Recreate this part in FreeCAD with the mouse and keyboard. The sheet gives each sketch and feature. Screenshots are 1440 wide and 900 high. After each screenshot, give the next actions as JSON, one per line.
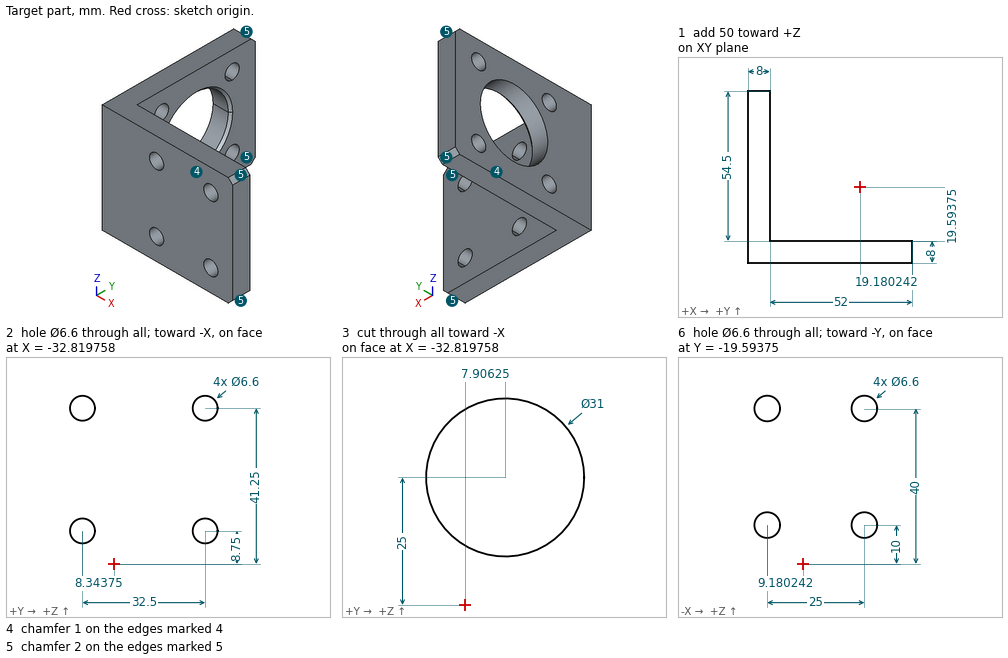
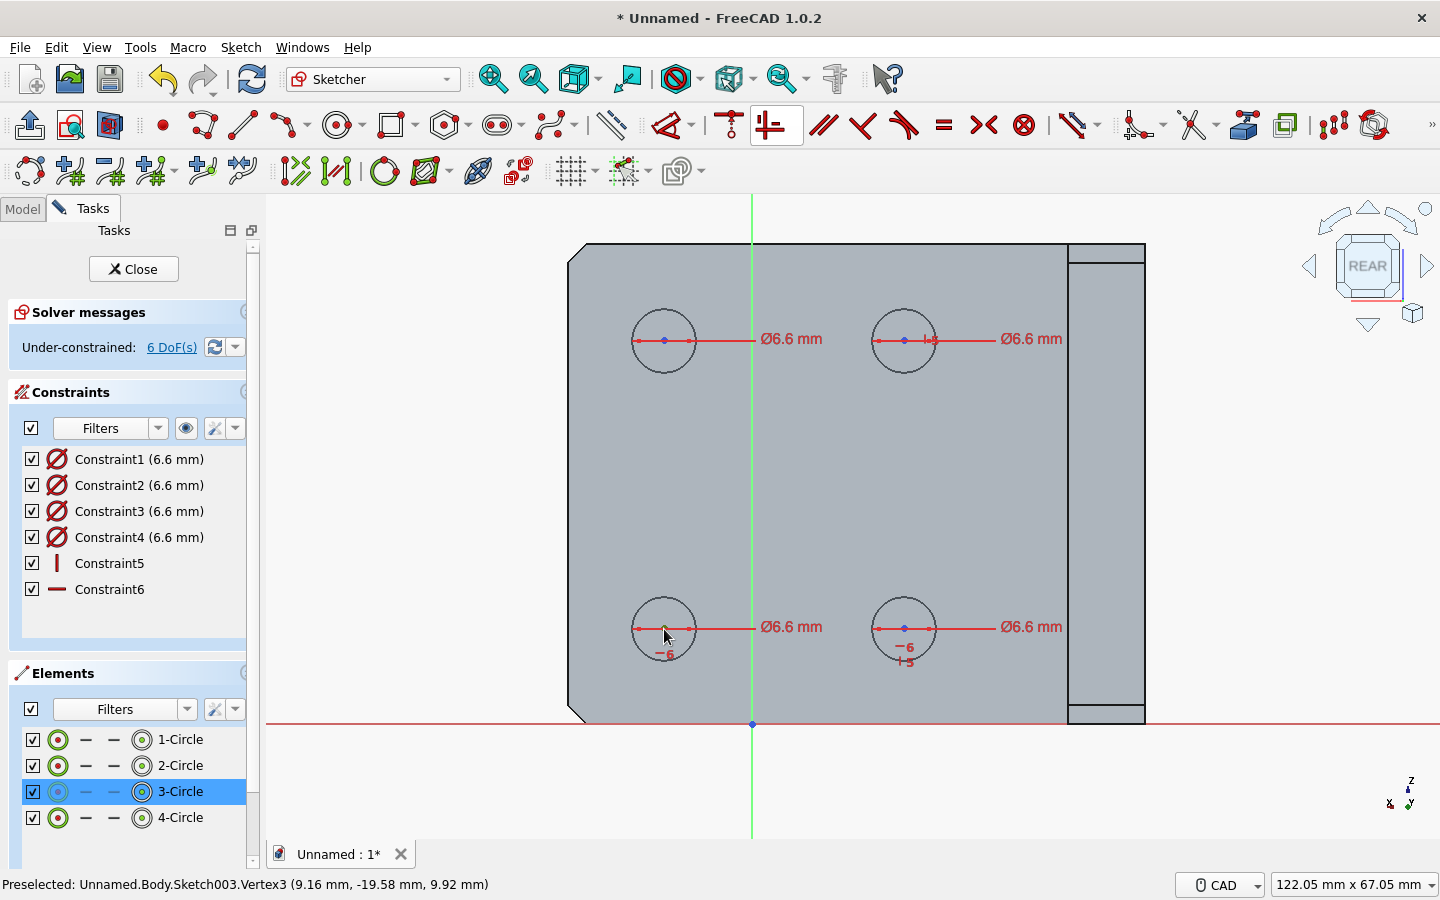
{"action": "left_click", "coordinate": [664, 341]}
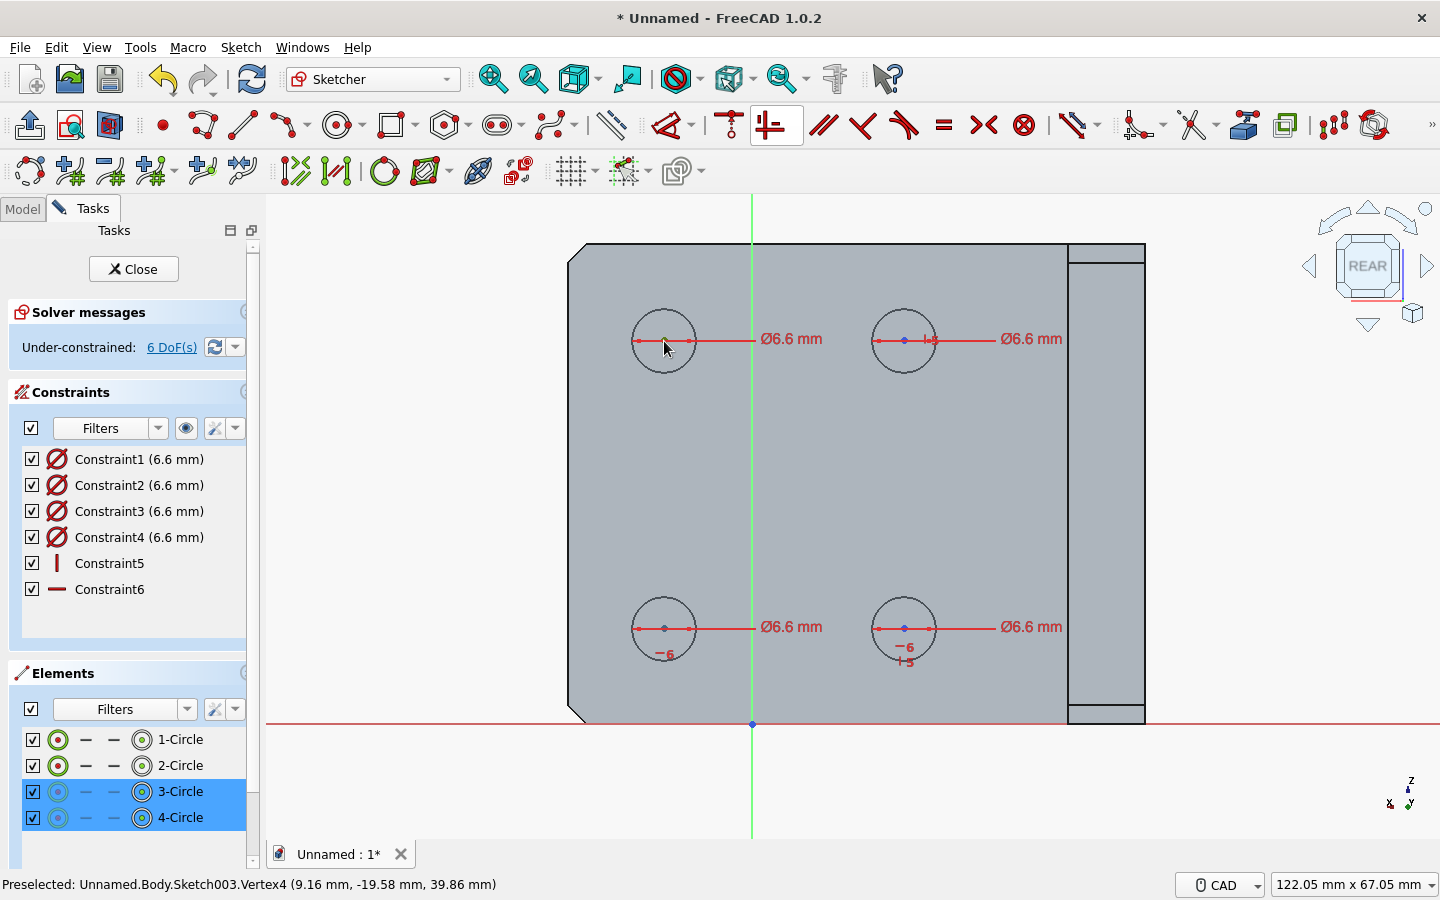
{"action": "left_click", "coordinate": [798, 126]}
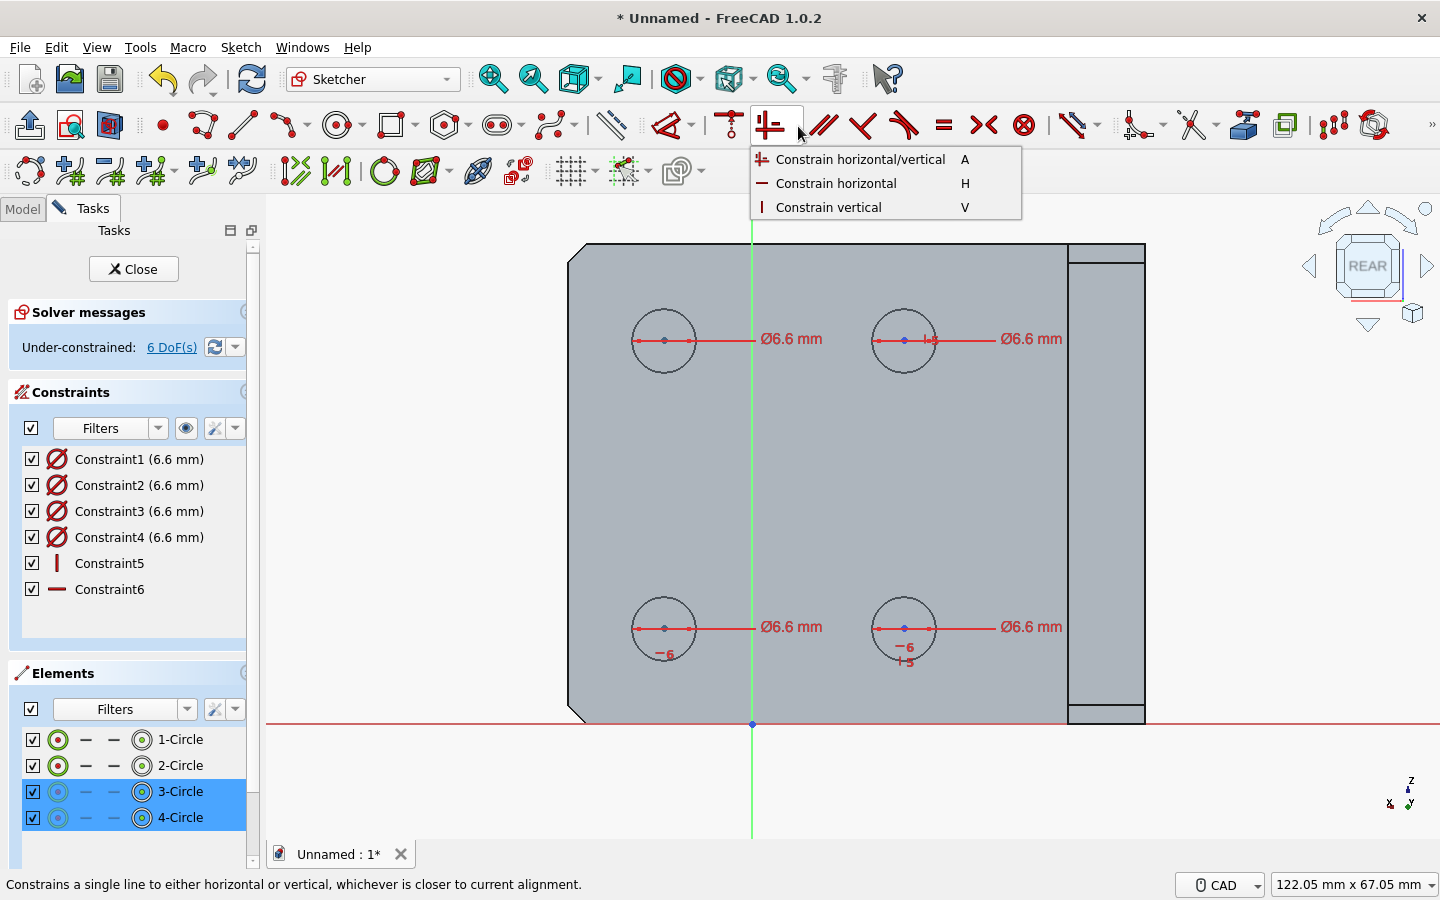
{"action": "left_click", "coordinate": [886, 207]}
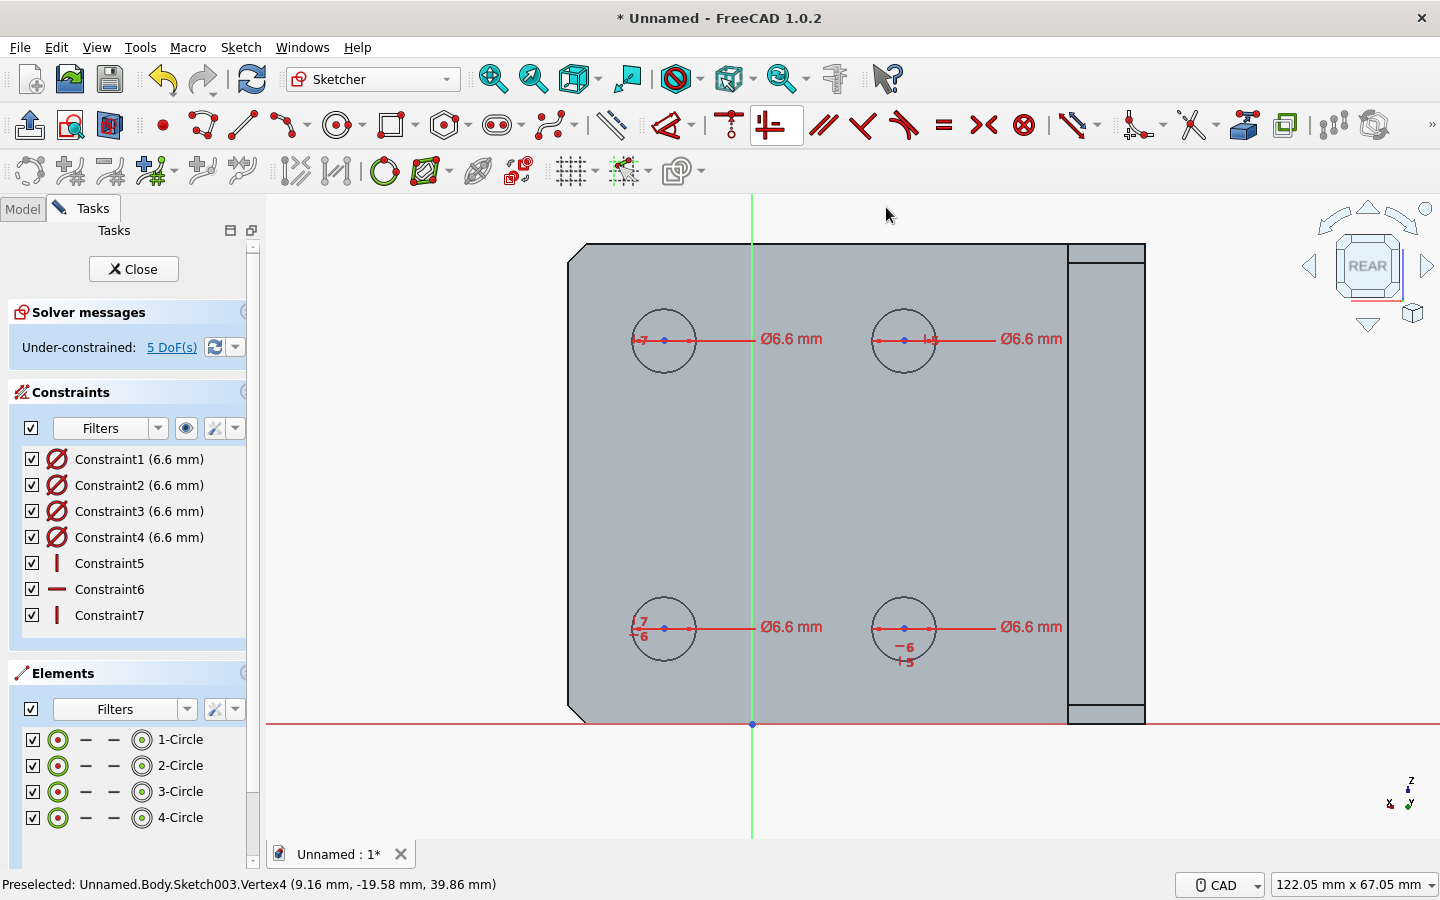
{"action": "left_click", "coordinate": [904, 341]}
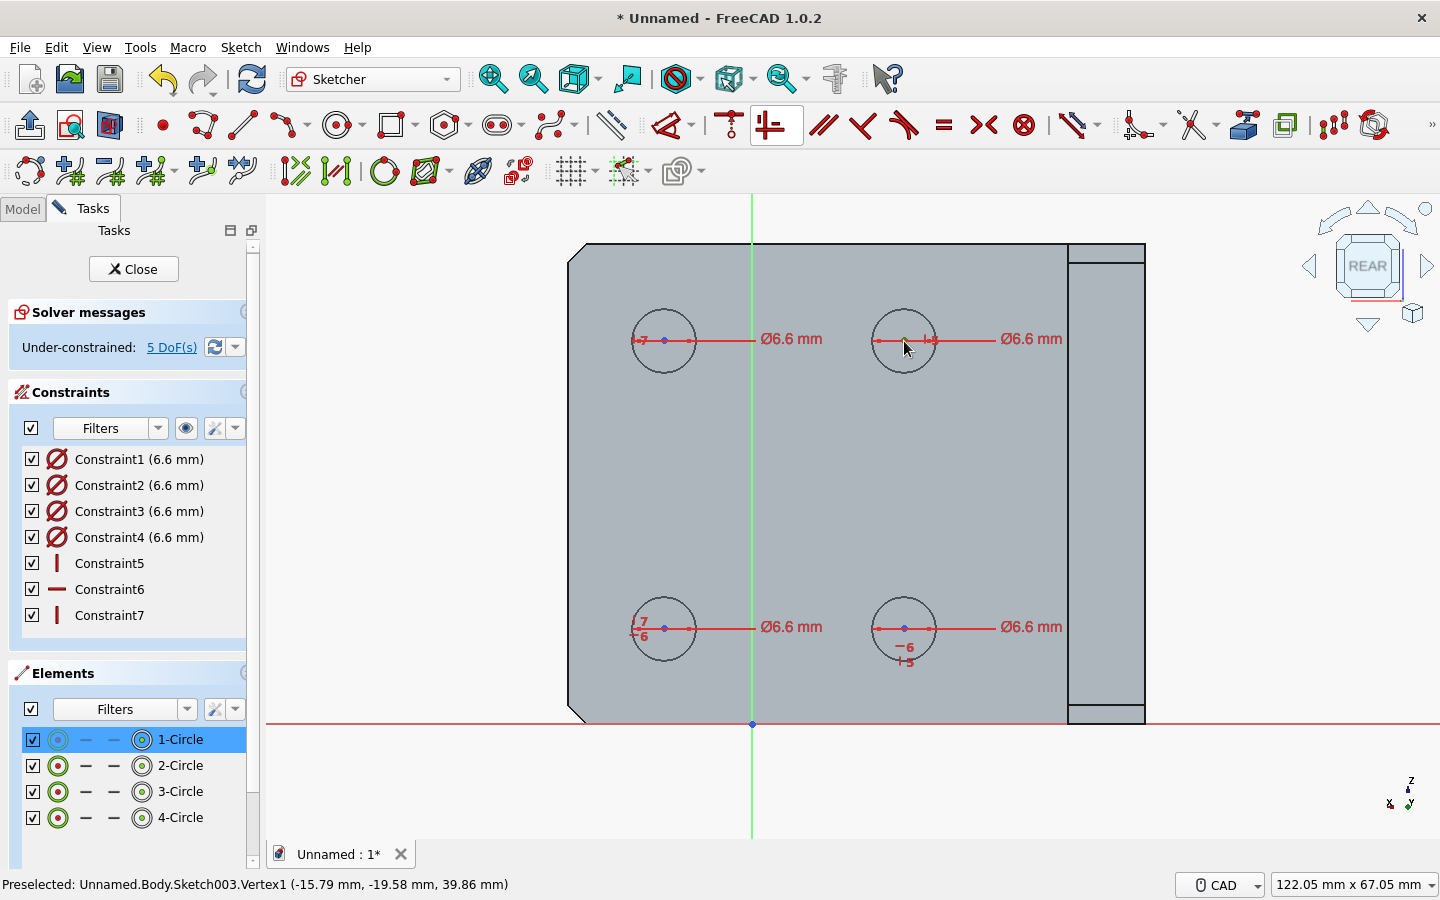
{"action": "left_click", "coordinate": [664, 341]}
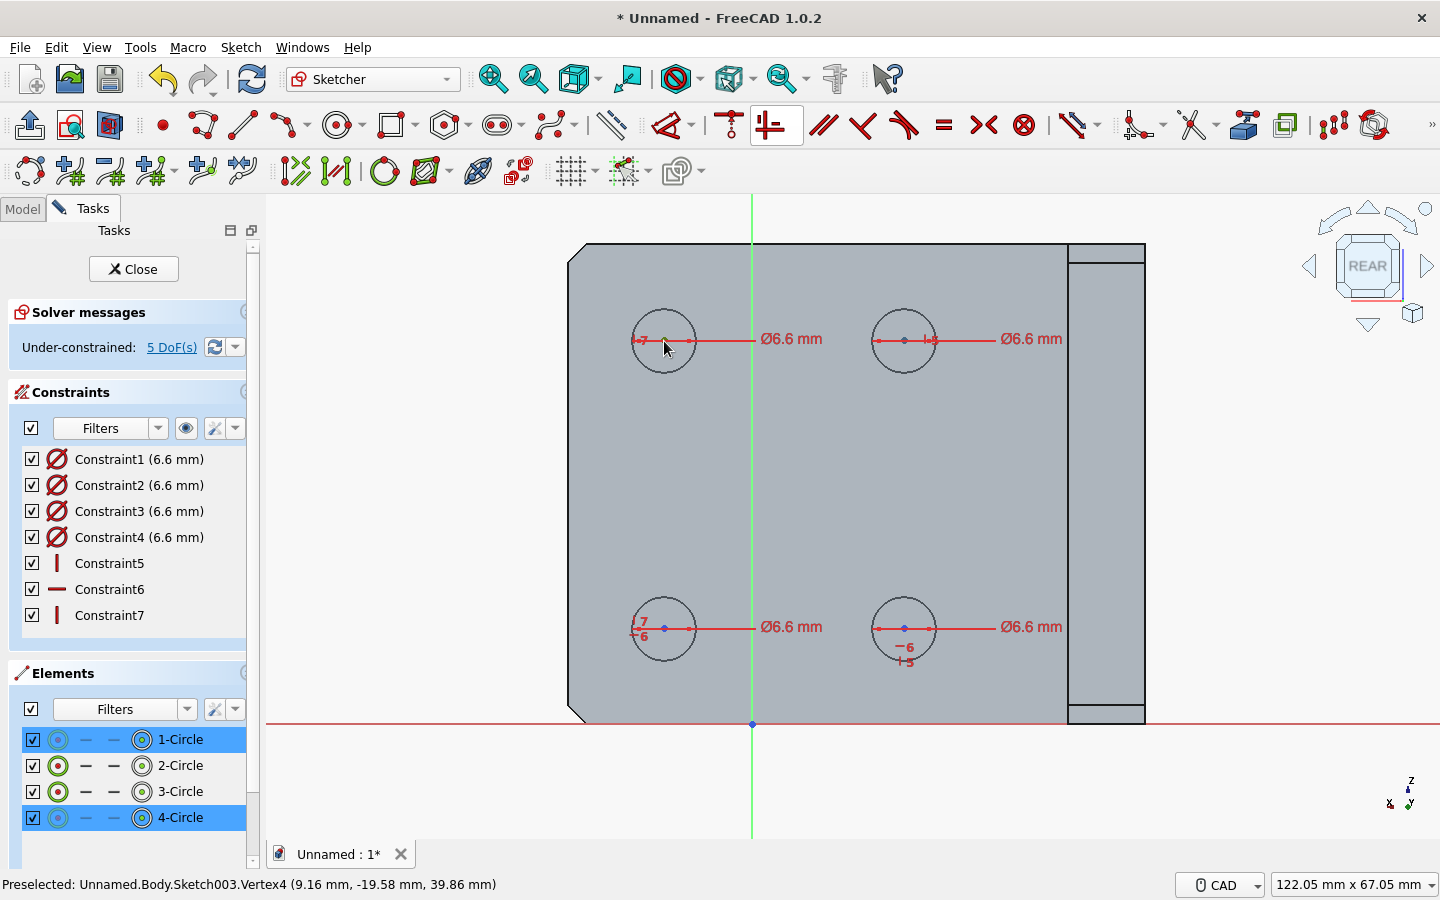
{"action": "left_click", "coordinate": [798, 126]}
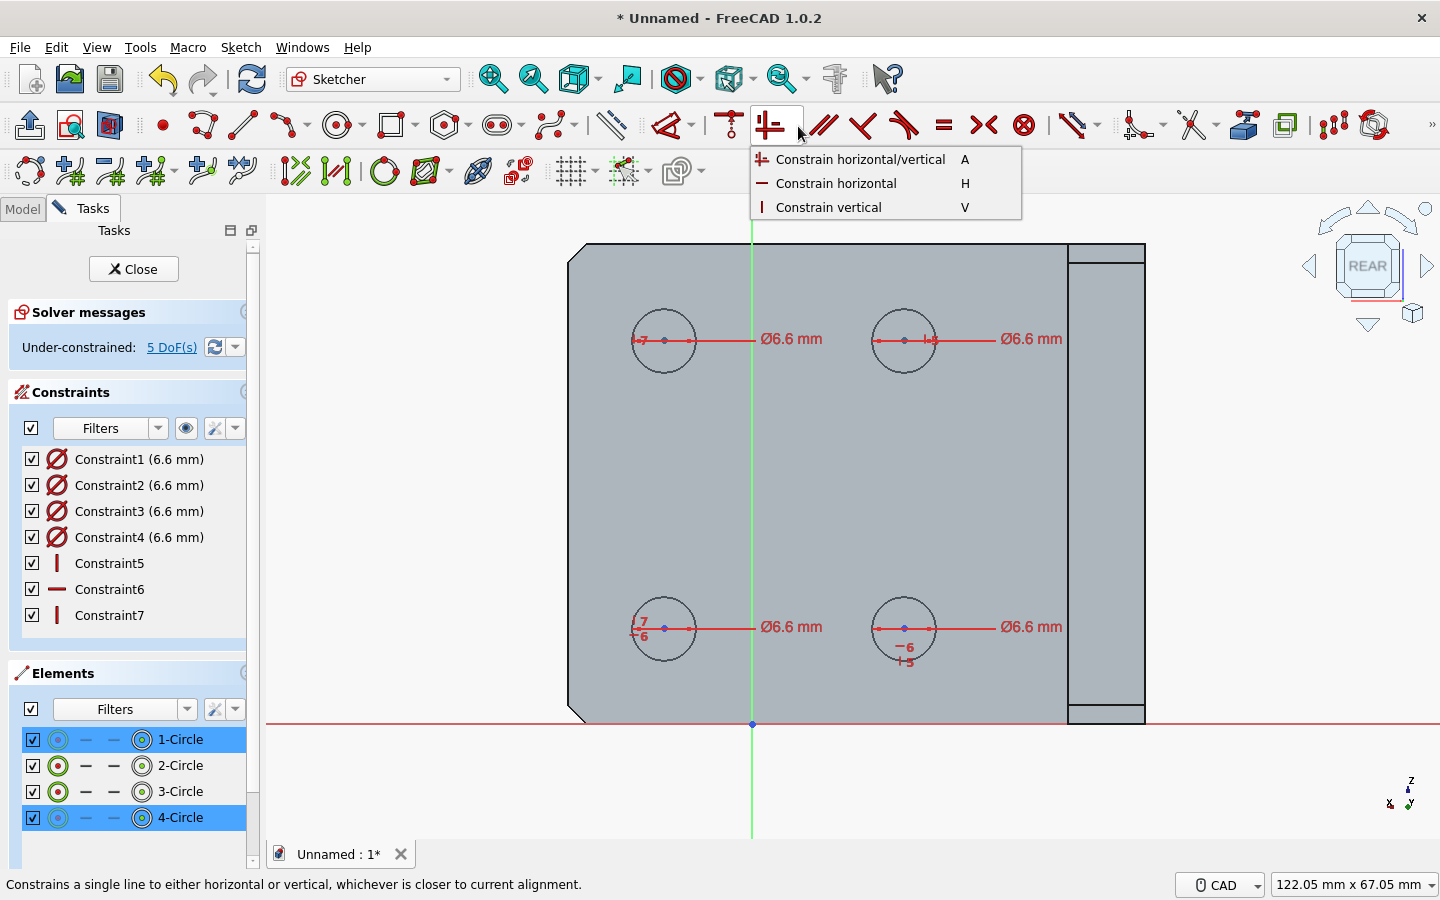
{"action": "left_click", "coordinate": [886, 183]}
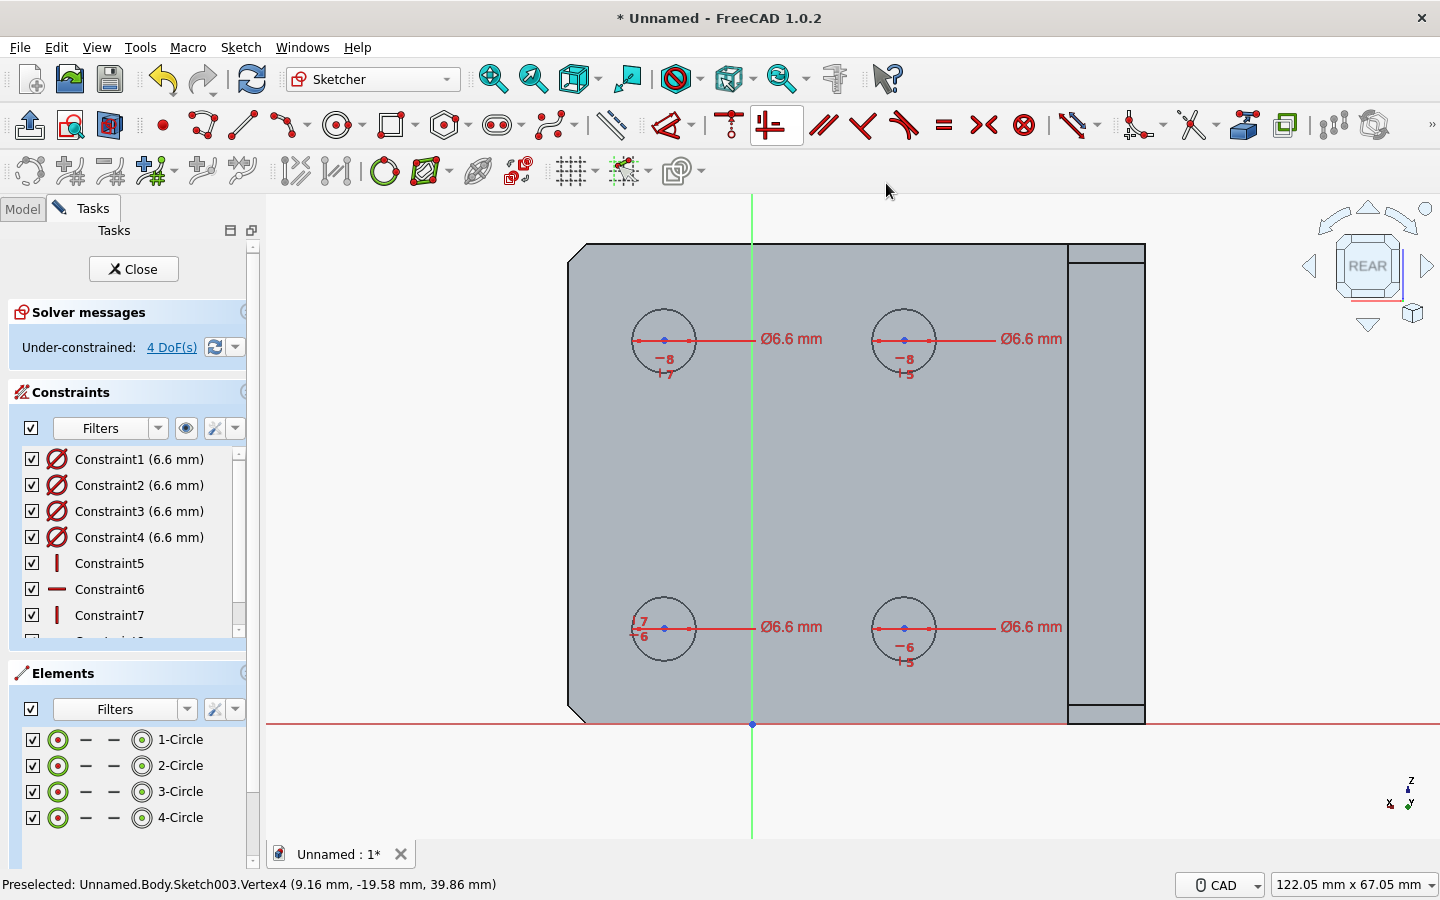
{"action": "left_click", "coordinate": [666, 126]}